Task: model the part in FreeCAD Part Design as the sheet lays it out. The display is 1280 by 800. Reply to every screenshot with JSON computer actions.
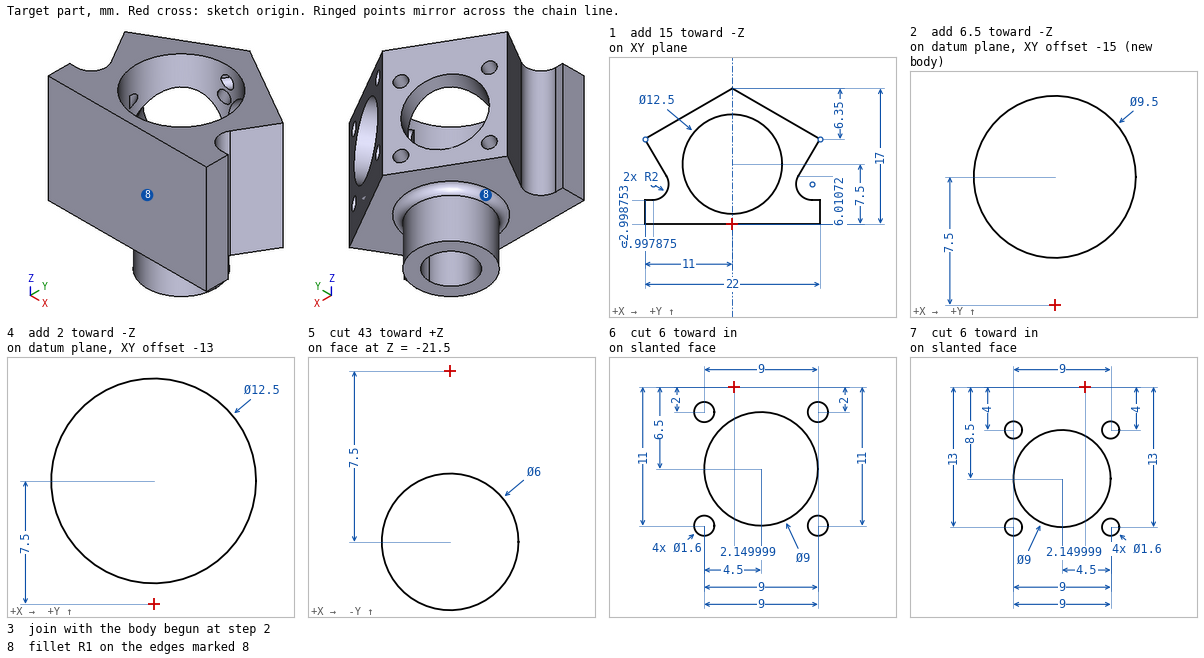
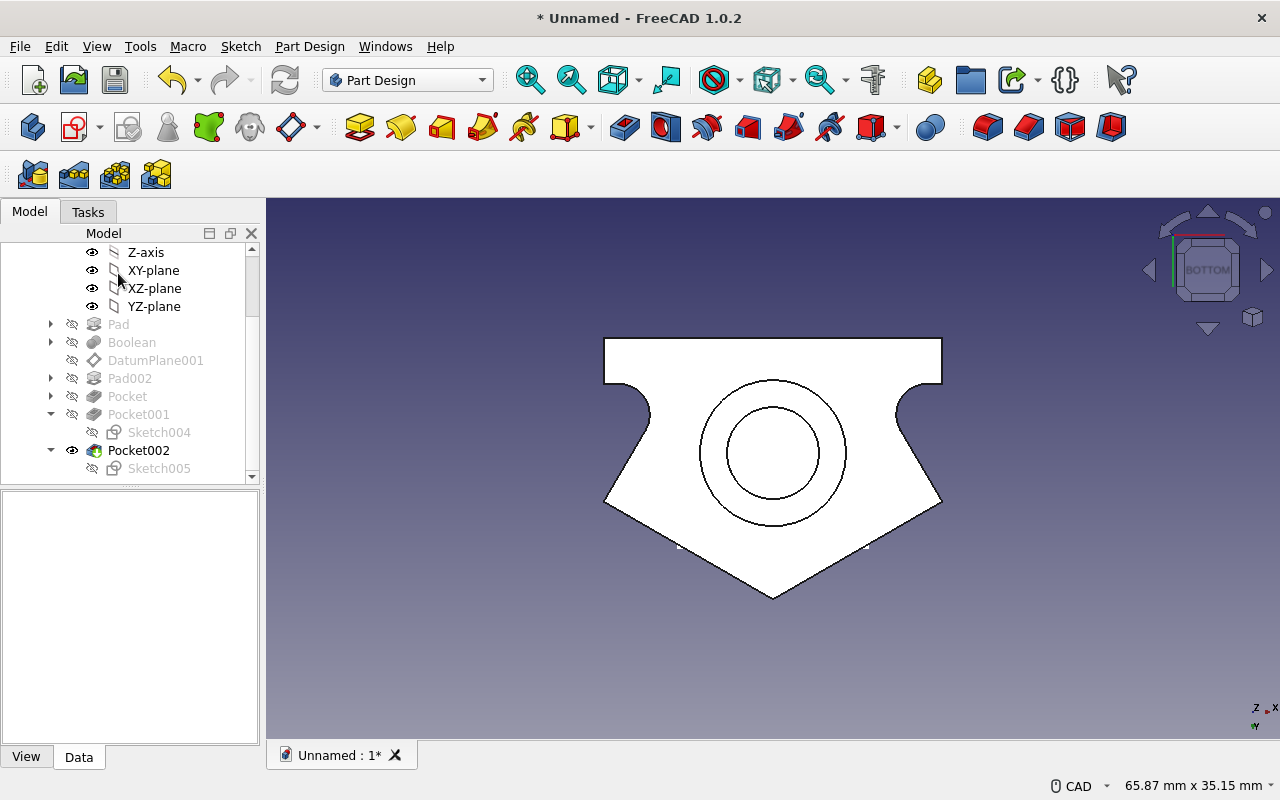
{"action": "key", "text": "4"}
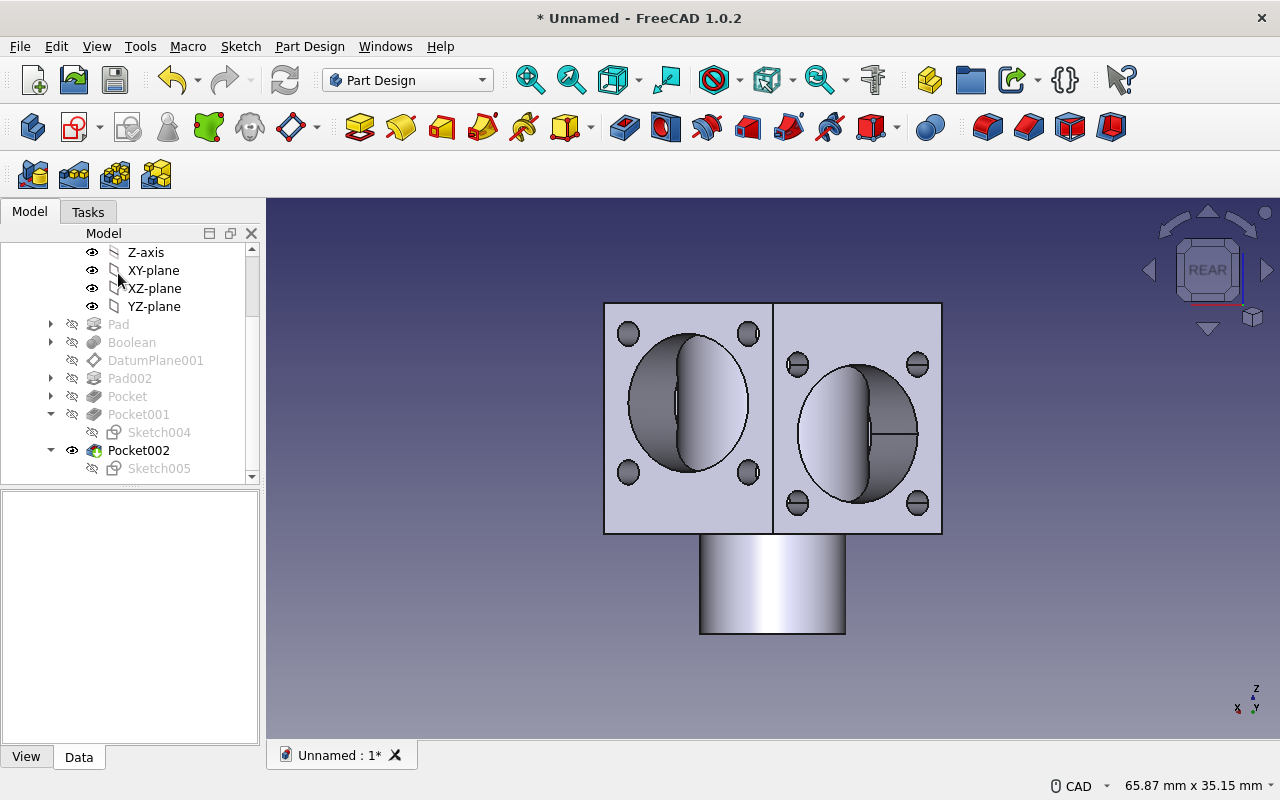
{"action": "key", "text": "6"}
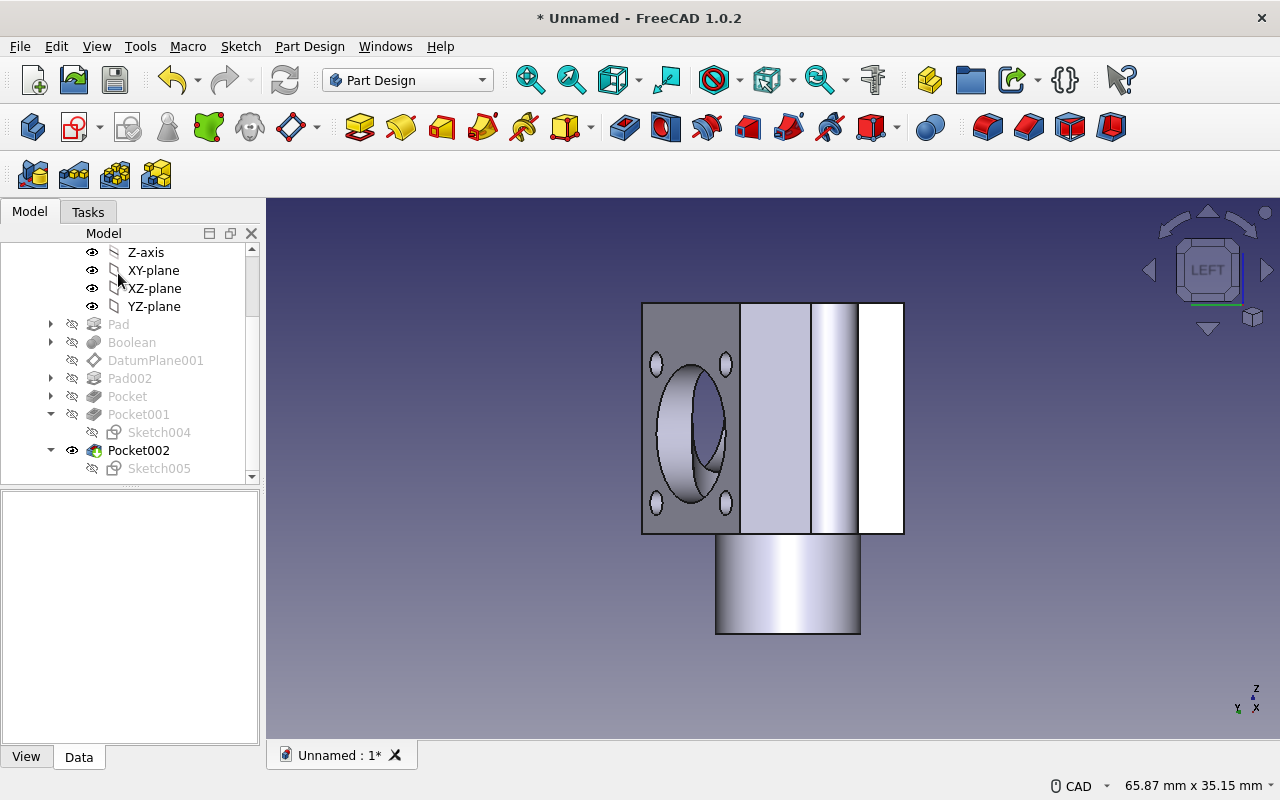
{"action": "key", "text": "v 3"}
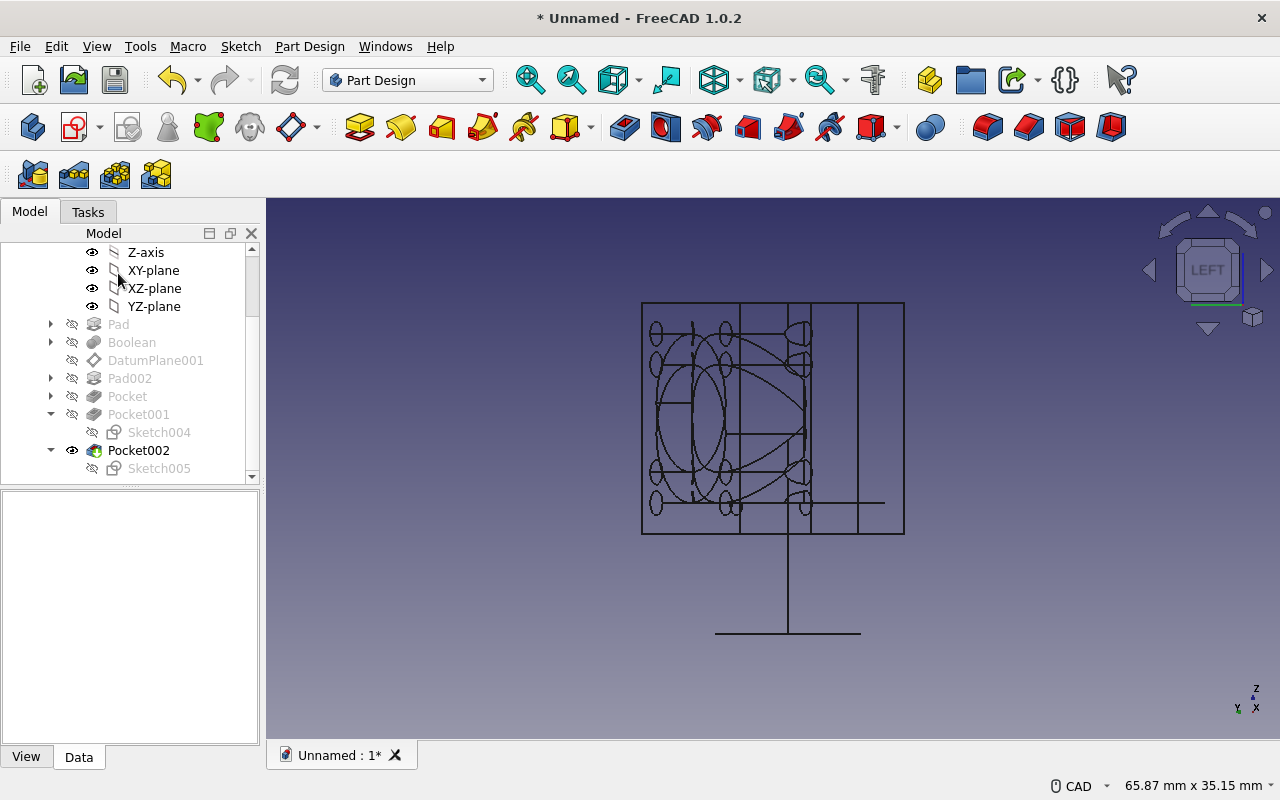
{"action": "key", "text": "0"}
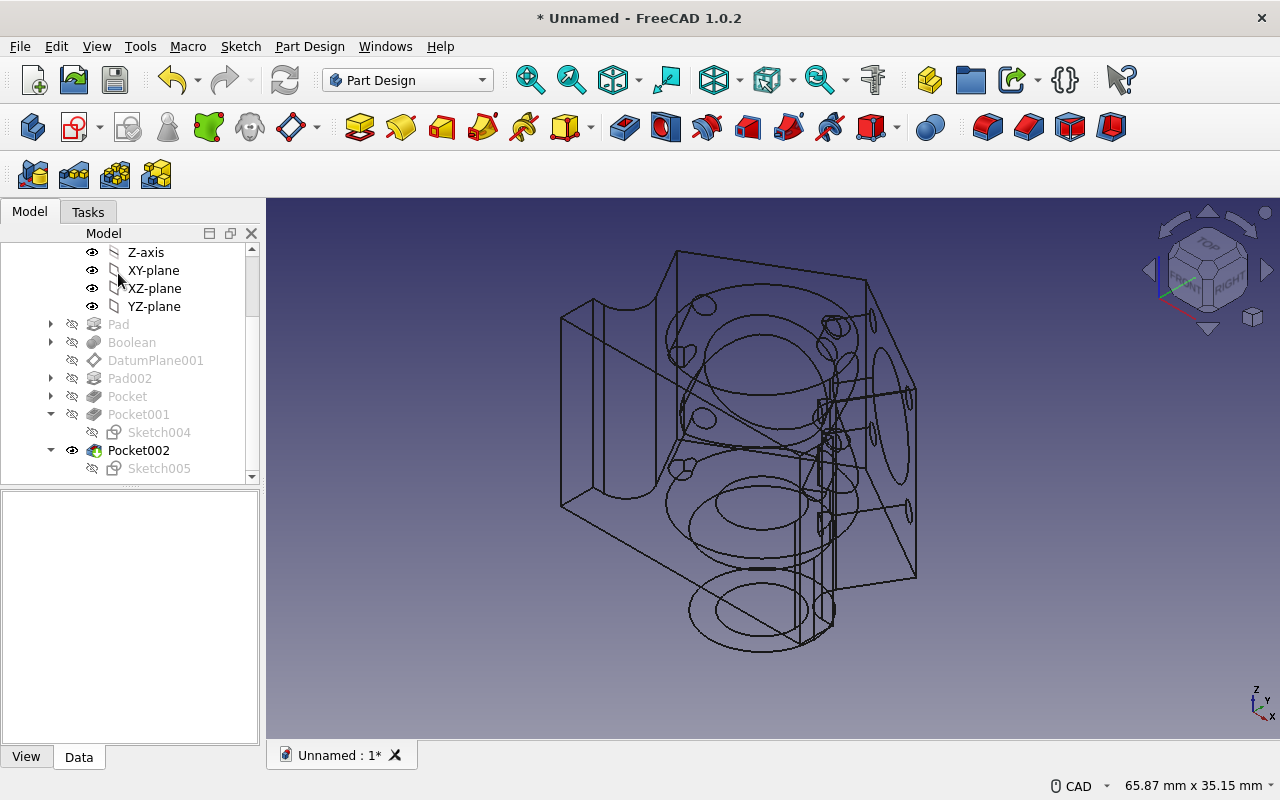
{"action": "left_click", "coordinate": [710, 497]}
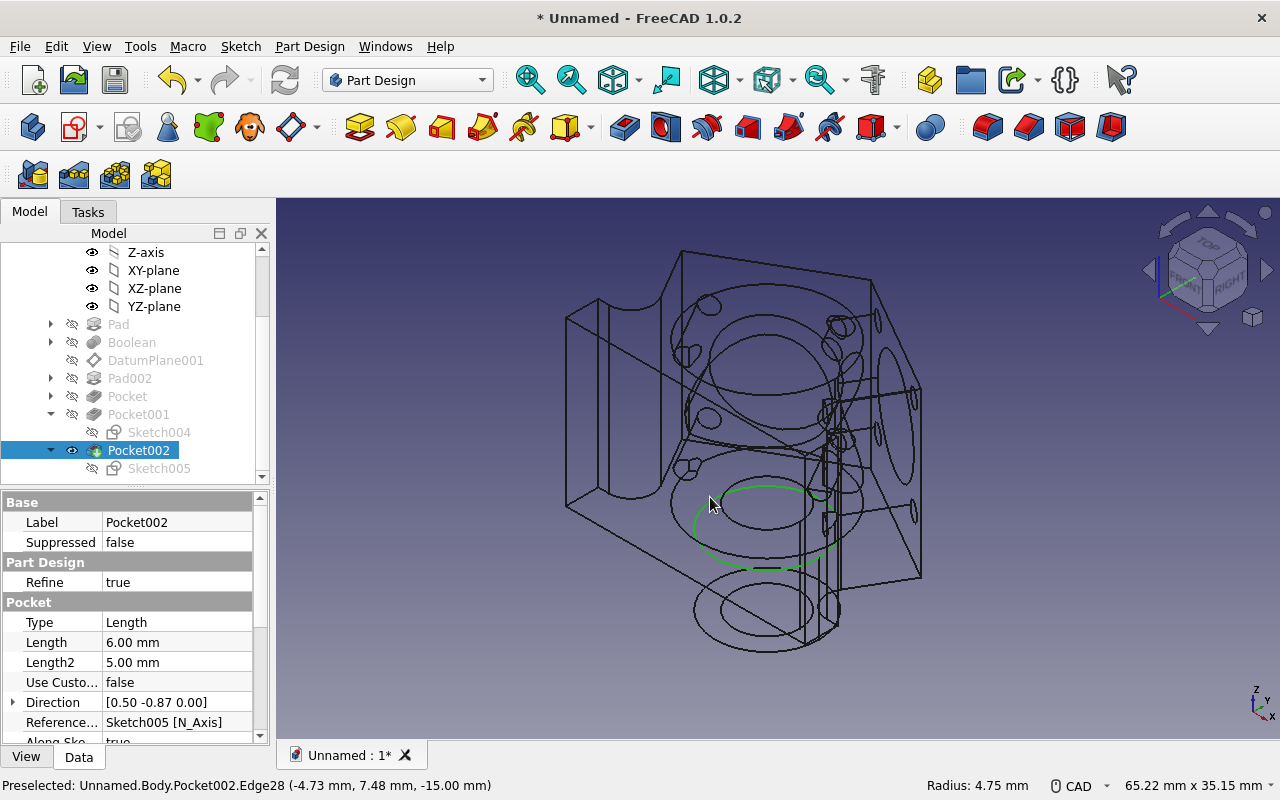
{"action": "key", "text": "v 1"}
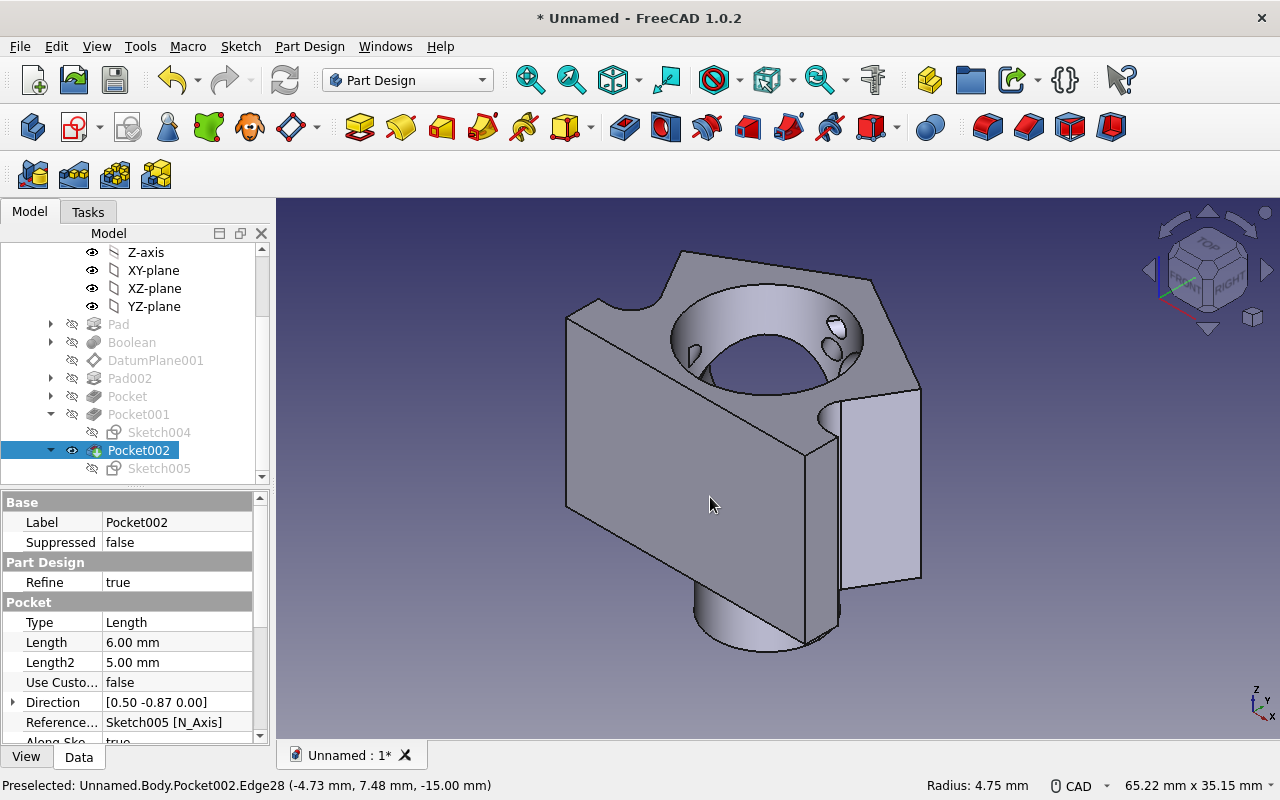
{"action": "left_click", "coordinate": [988, 128]}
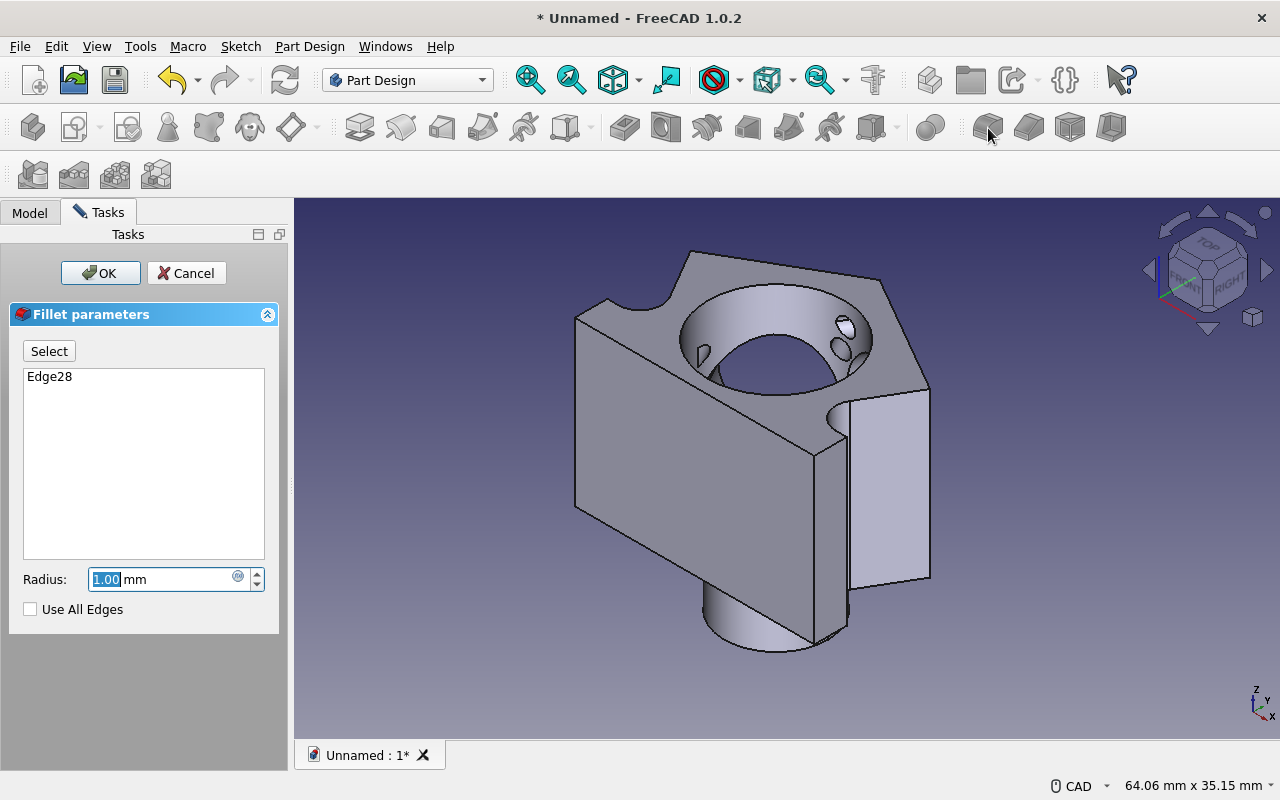
{"action": "type", "text": "1"}
{"action": "key", "text": "Tab"}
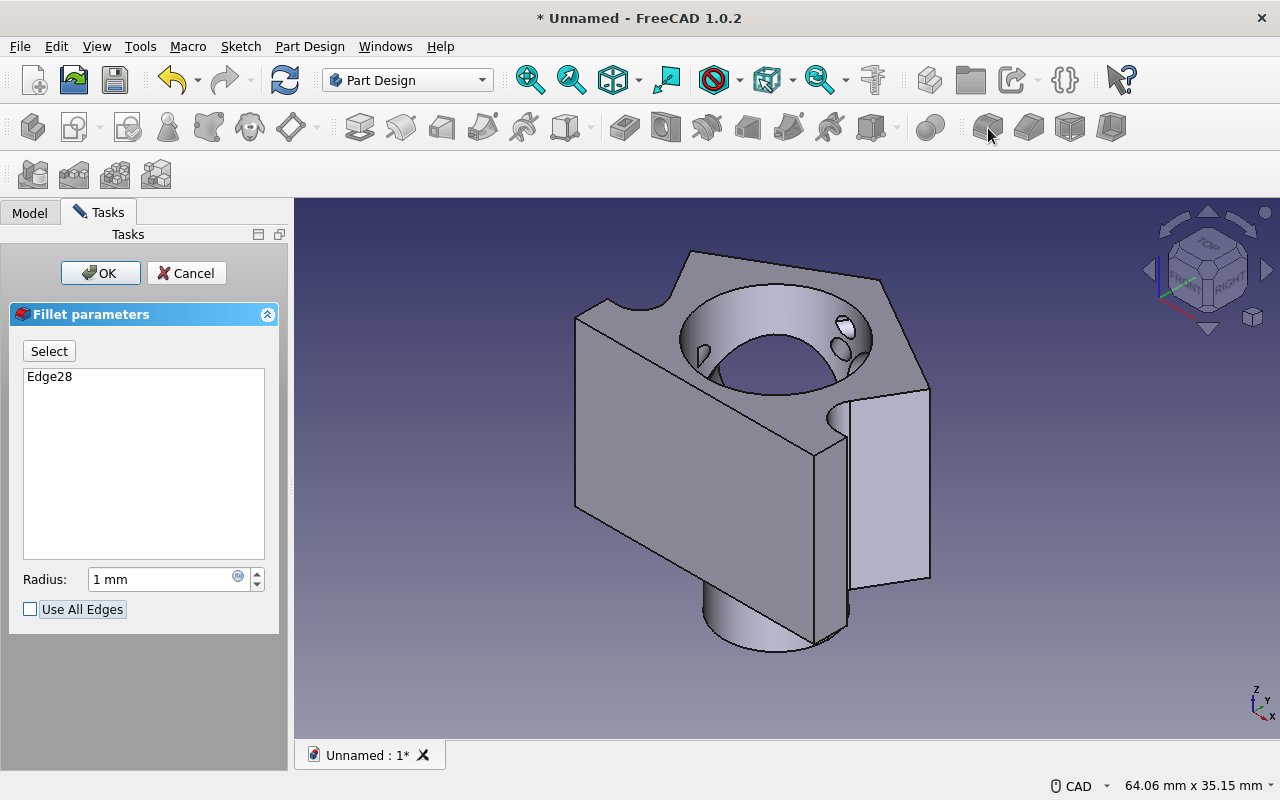
{"action": "left_click", "coordinate": [101, 273]}